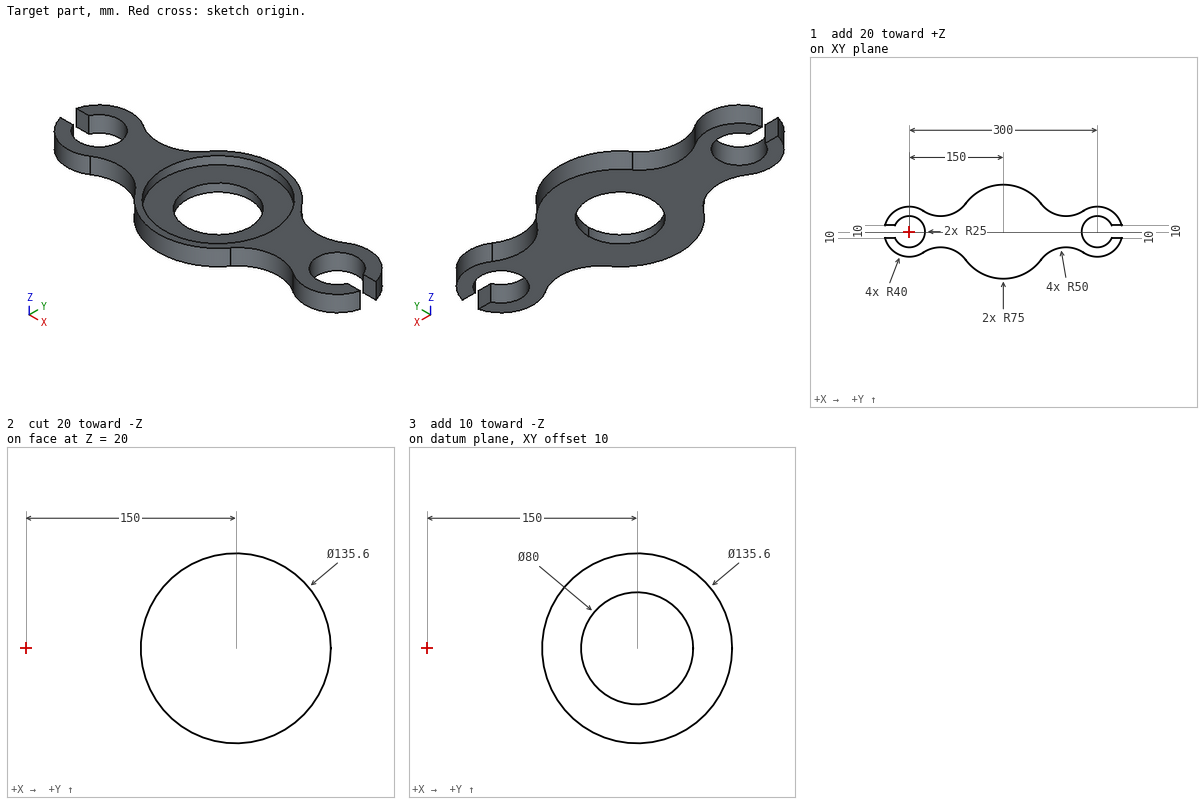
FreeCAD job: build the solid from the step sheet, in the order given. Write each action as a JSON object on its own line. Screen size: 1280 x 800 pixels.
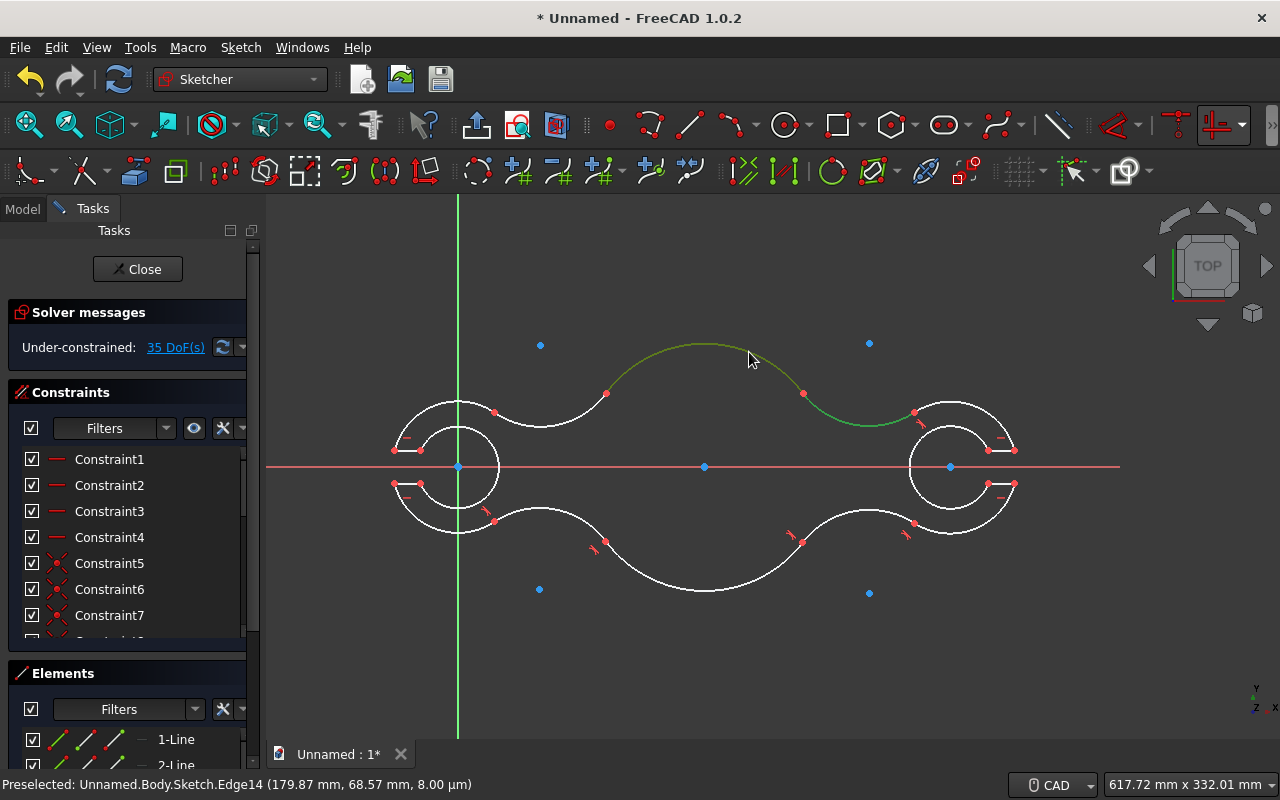
{"action": "key", "text": "t"}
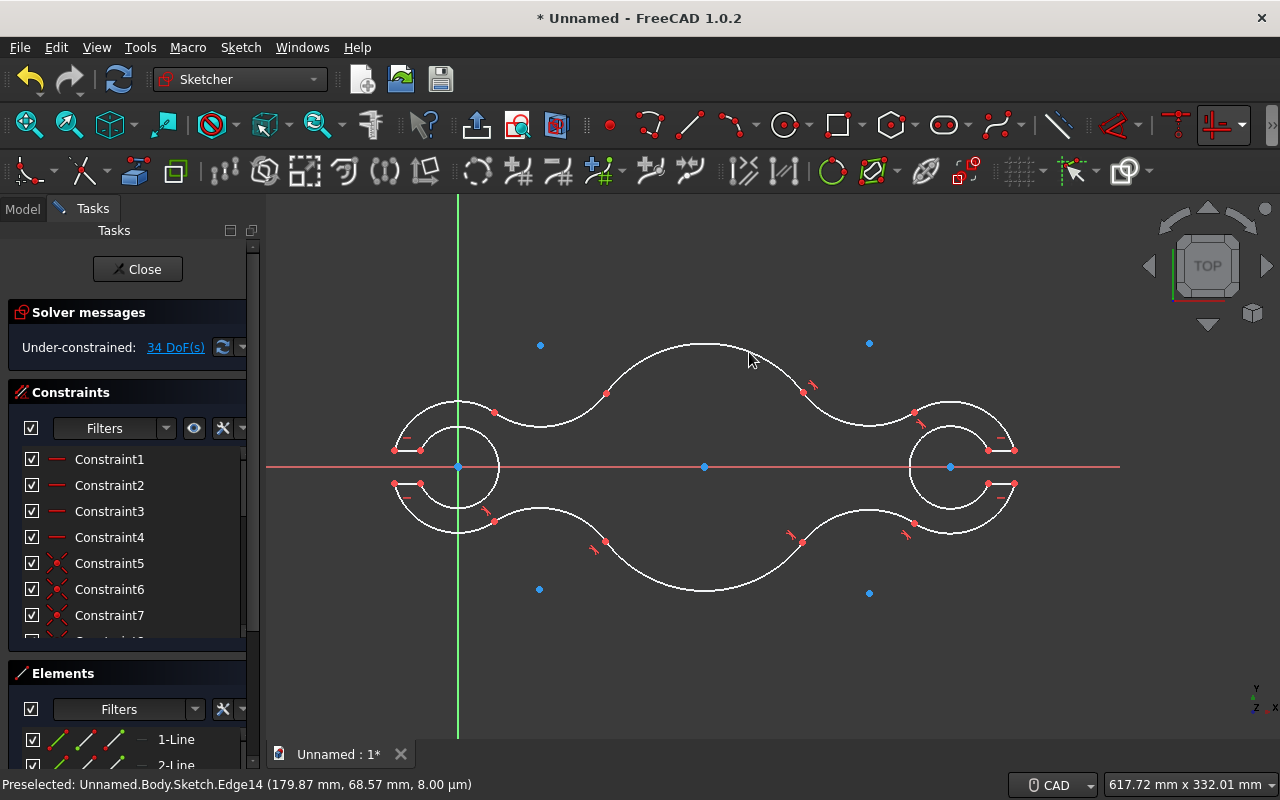
{"action": "left_click", "coordinate": [749, 352]}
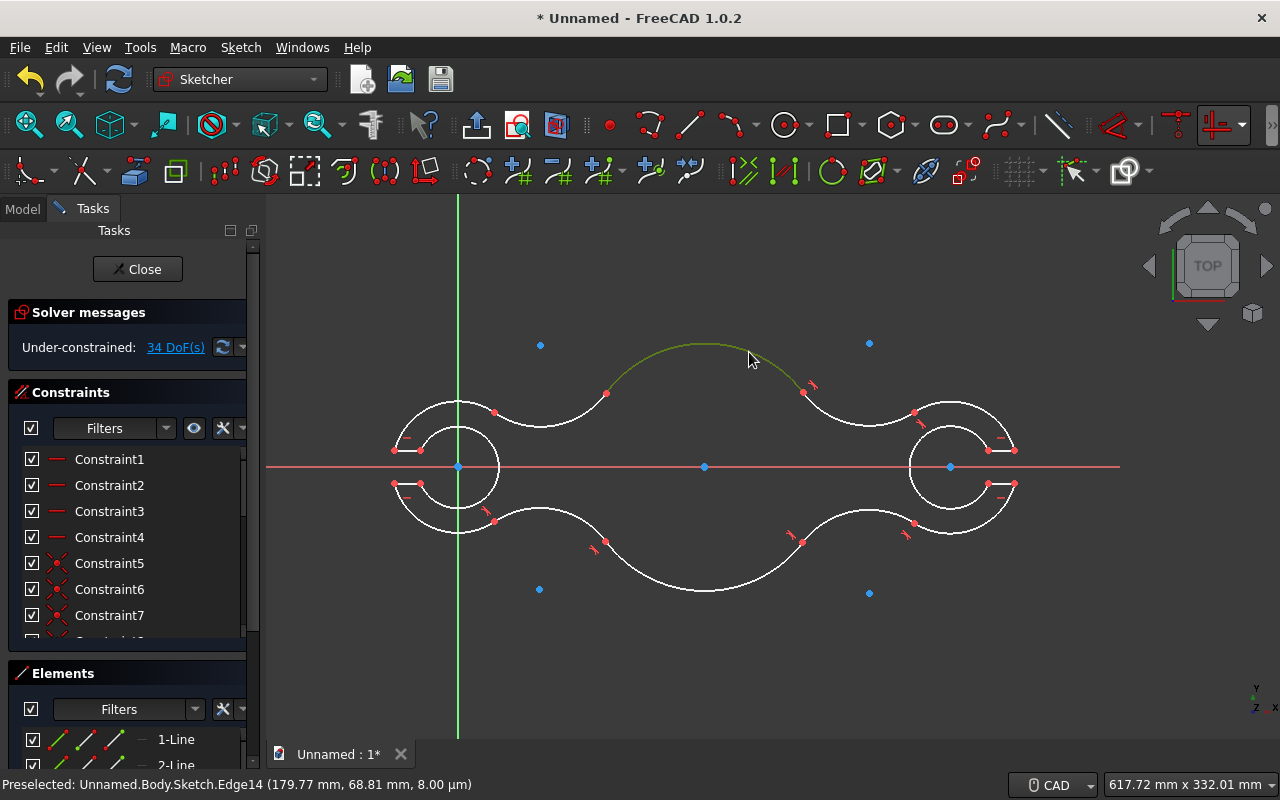
{"action": "left_click", "coordinate": [529, 426]}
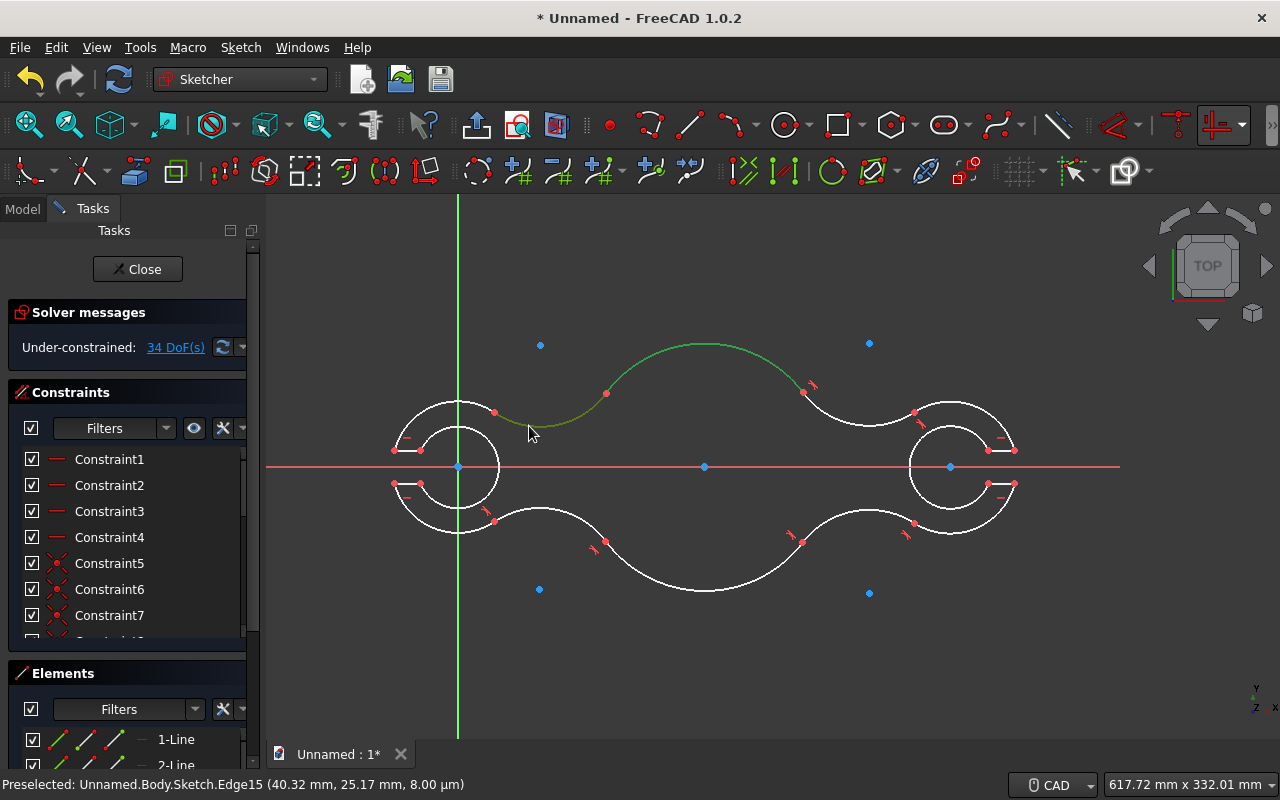
{"action": "key", "text": "t"}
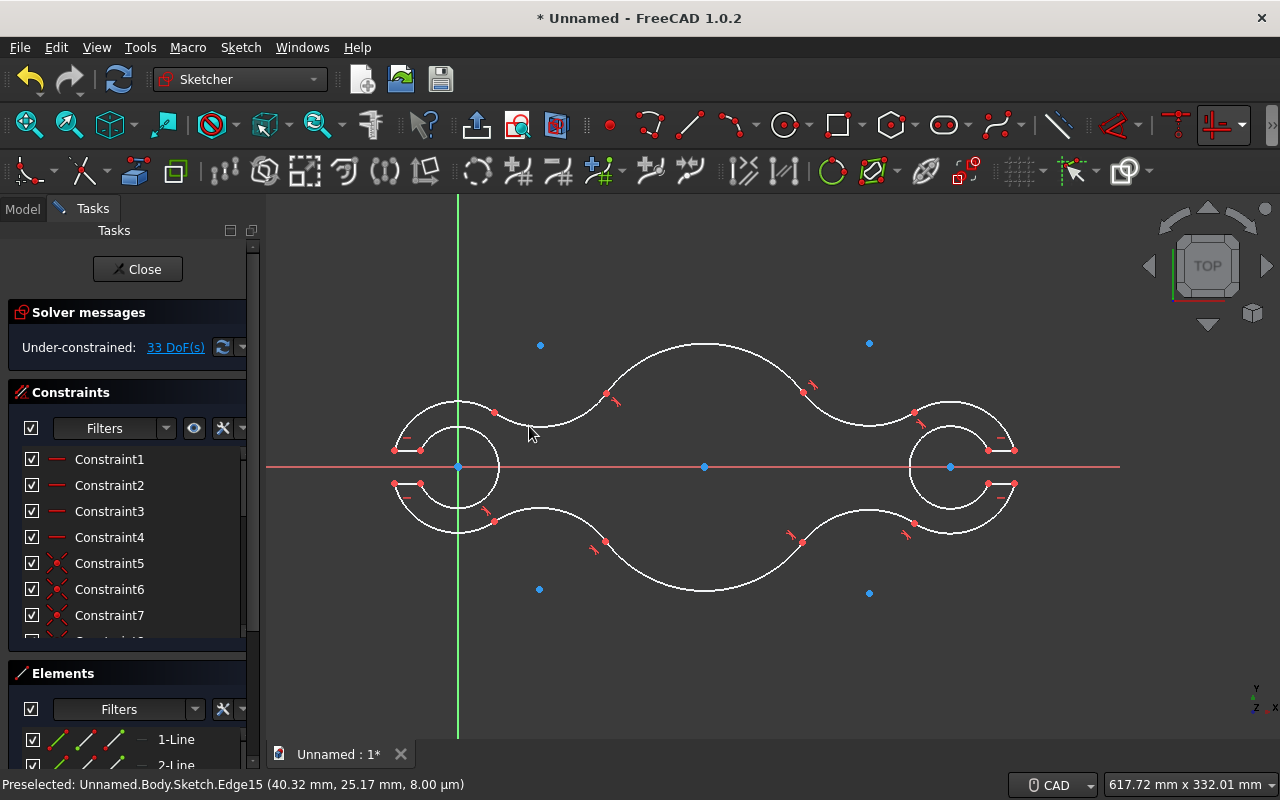
{"action": "left_click", "coordinate": [529, 426]}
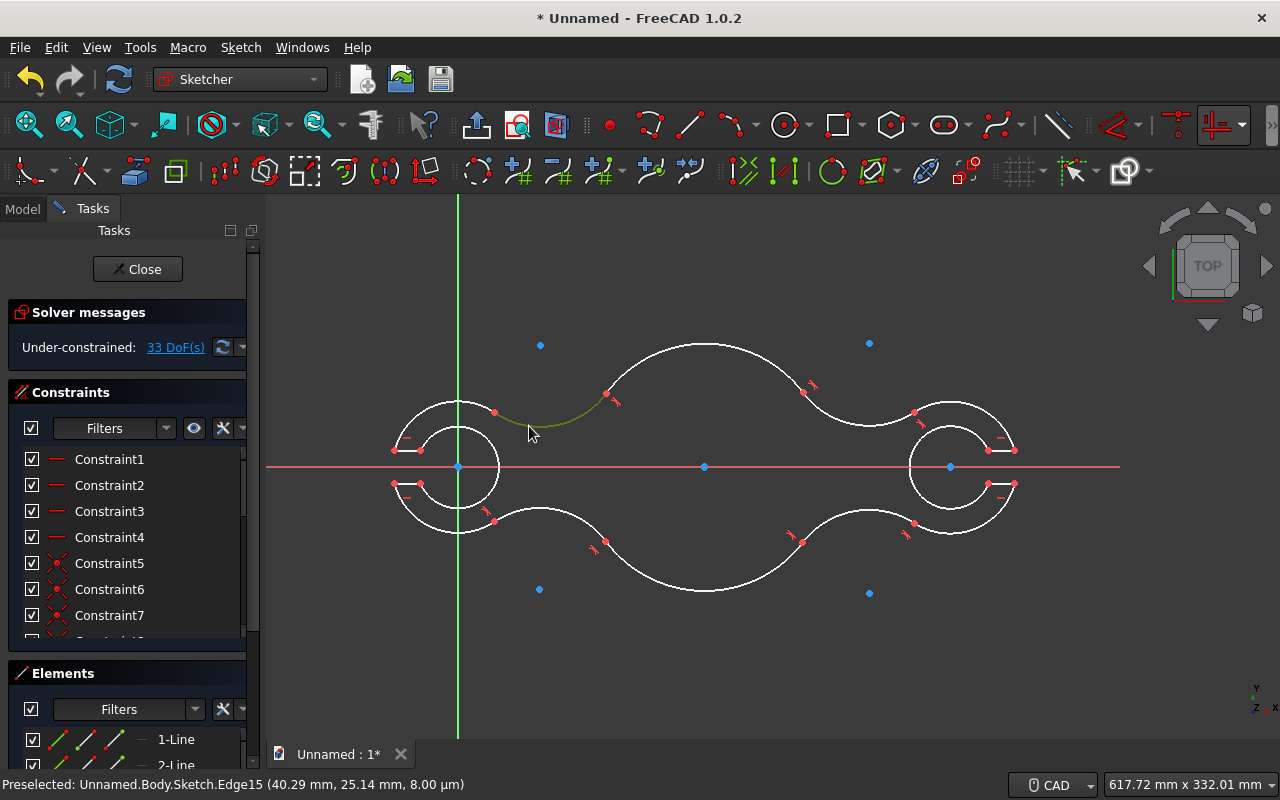
{"action": "left_click", "coordinate": [459, 401]}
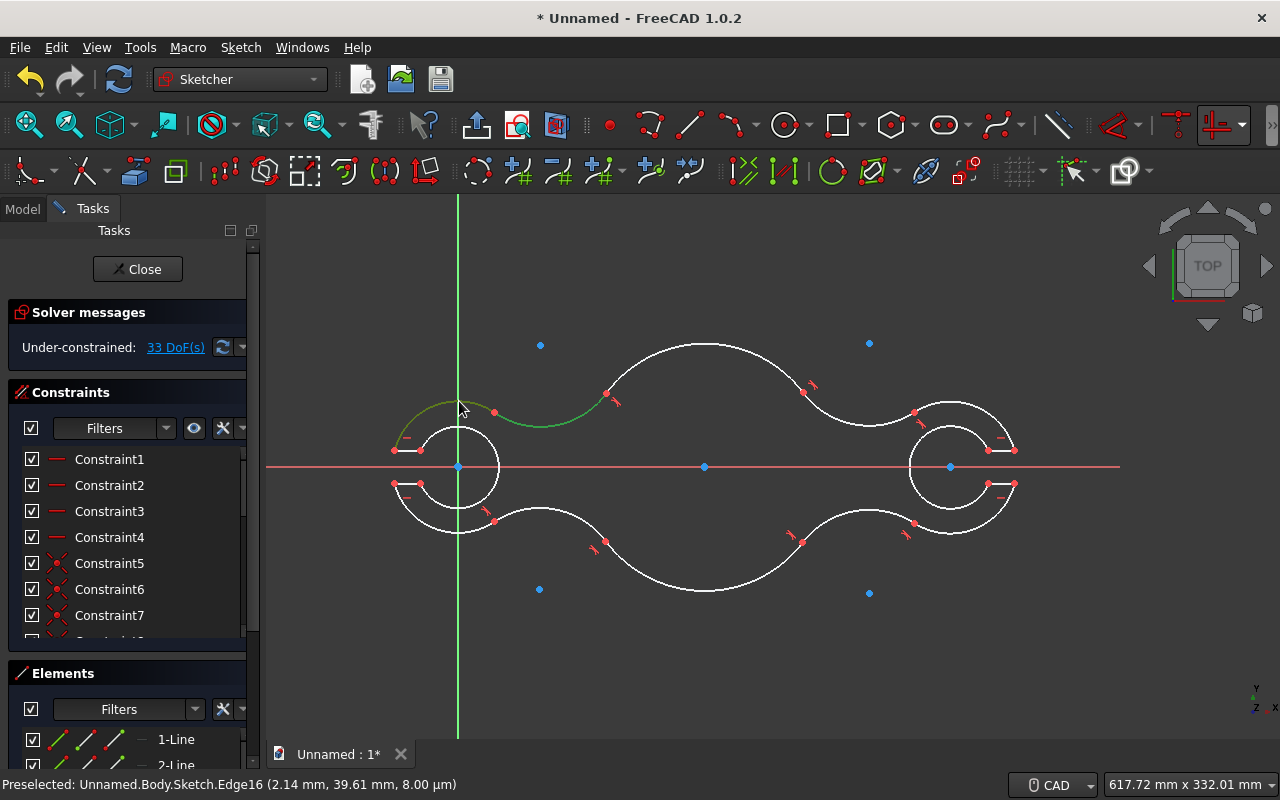
{"action": "key", "text": "t"}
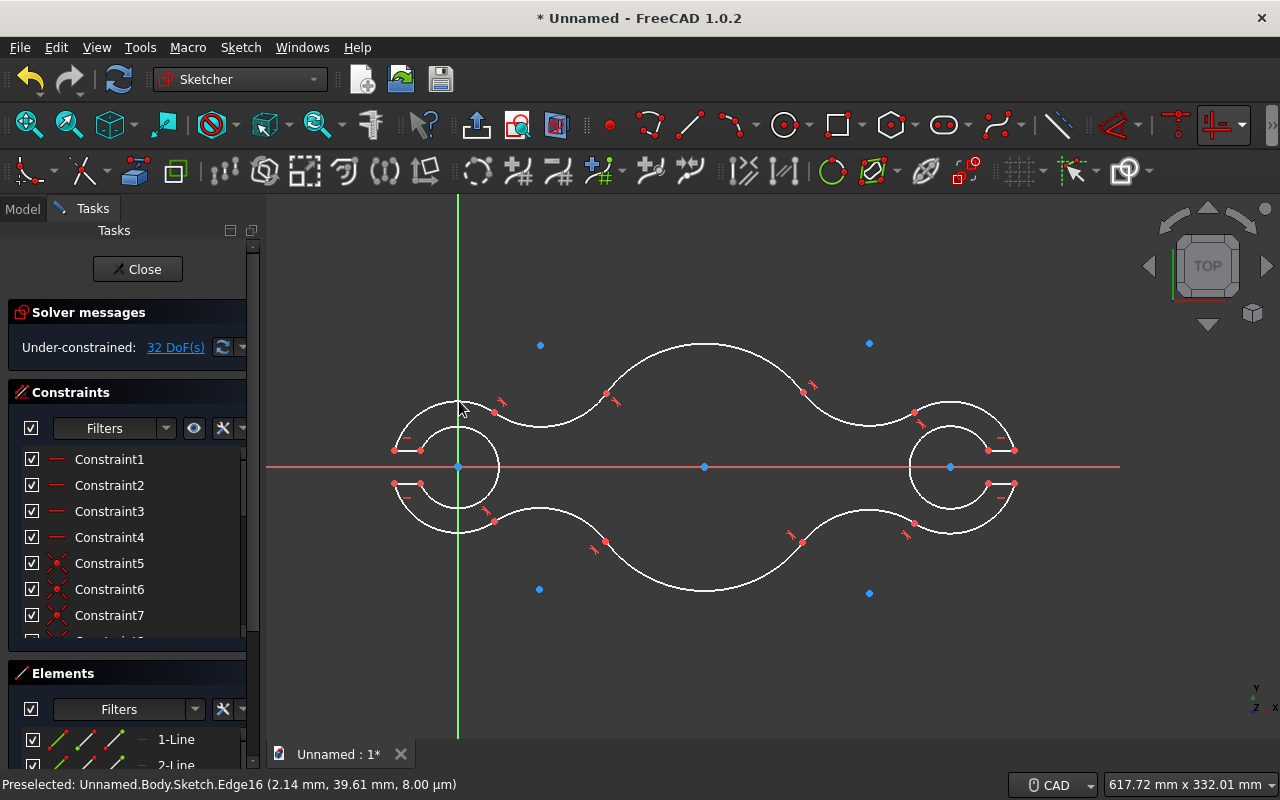
{"action": "left_click", "coordinate": [477, 504]}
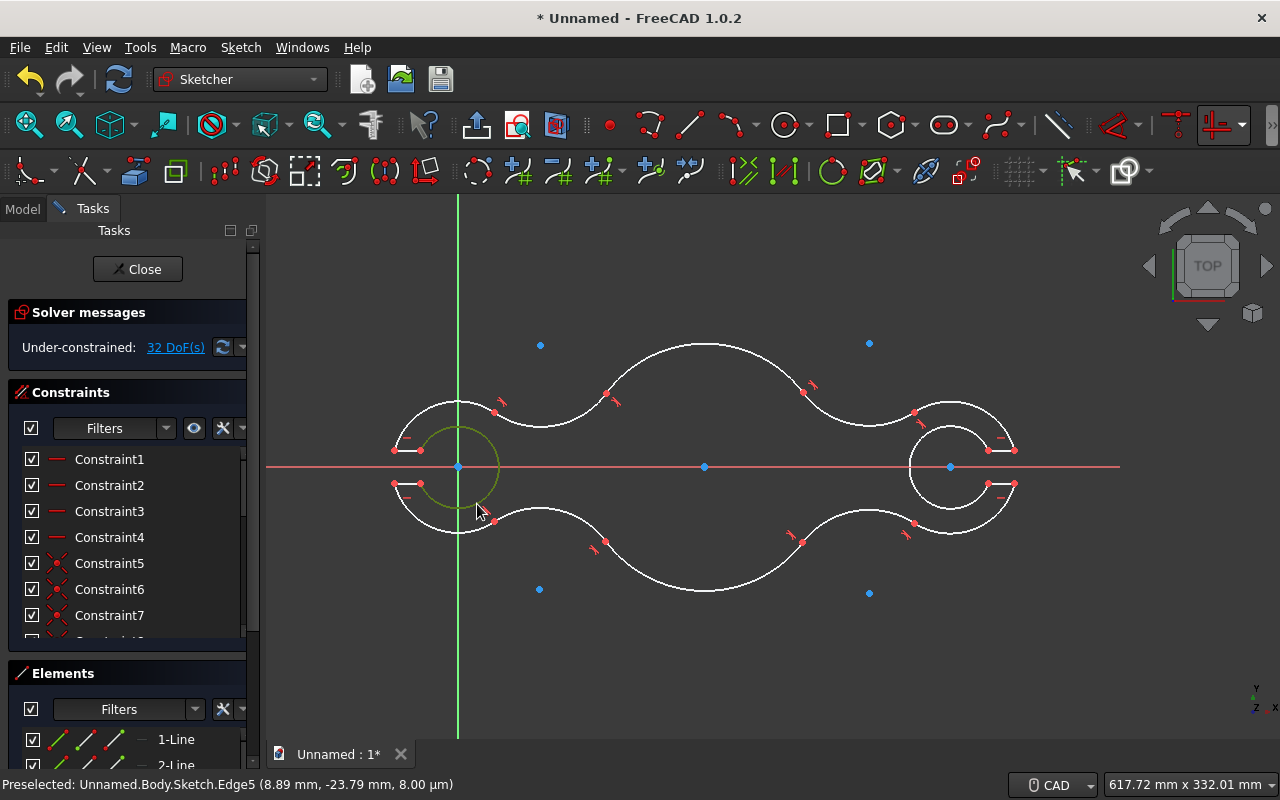
{"action": "left_click", "coordinate": [414, 516]}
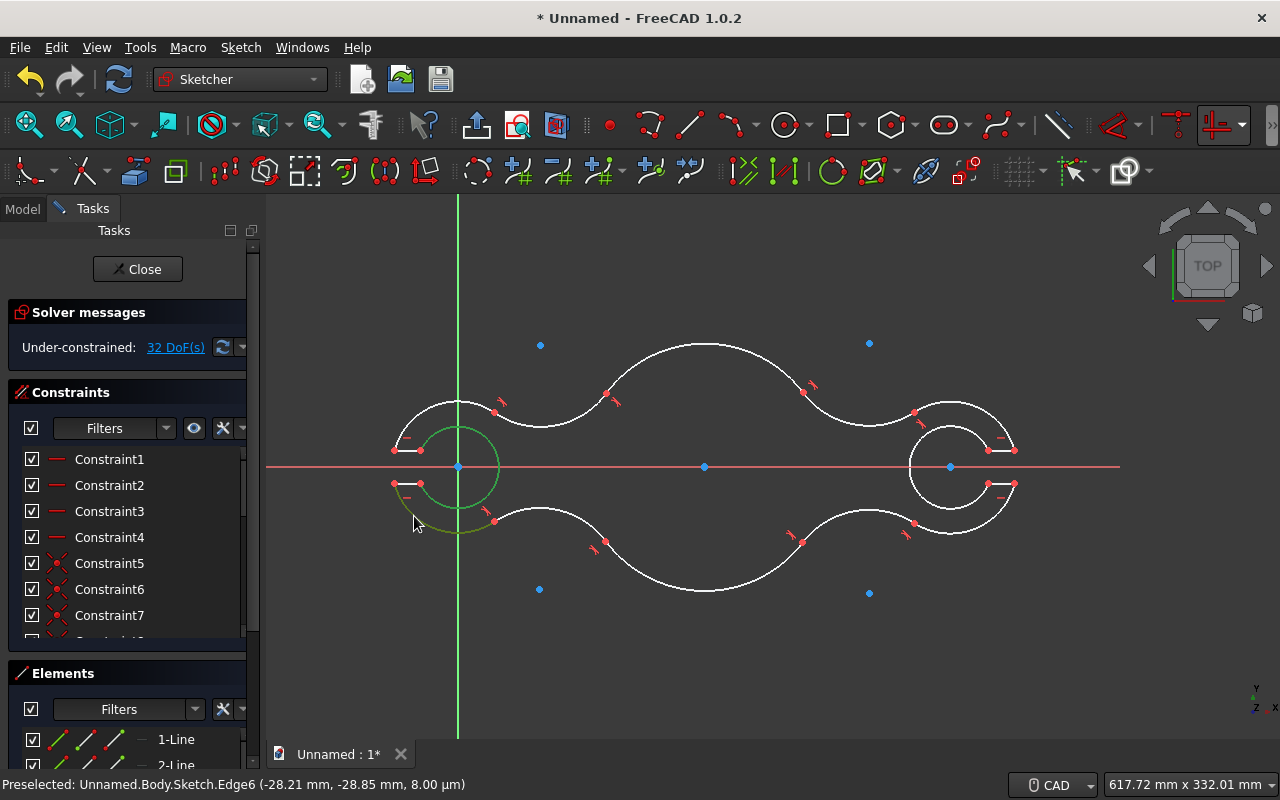
{"action": "left_click", "coordinate": [1176, 126]}